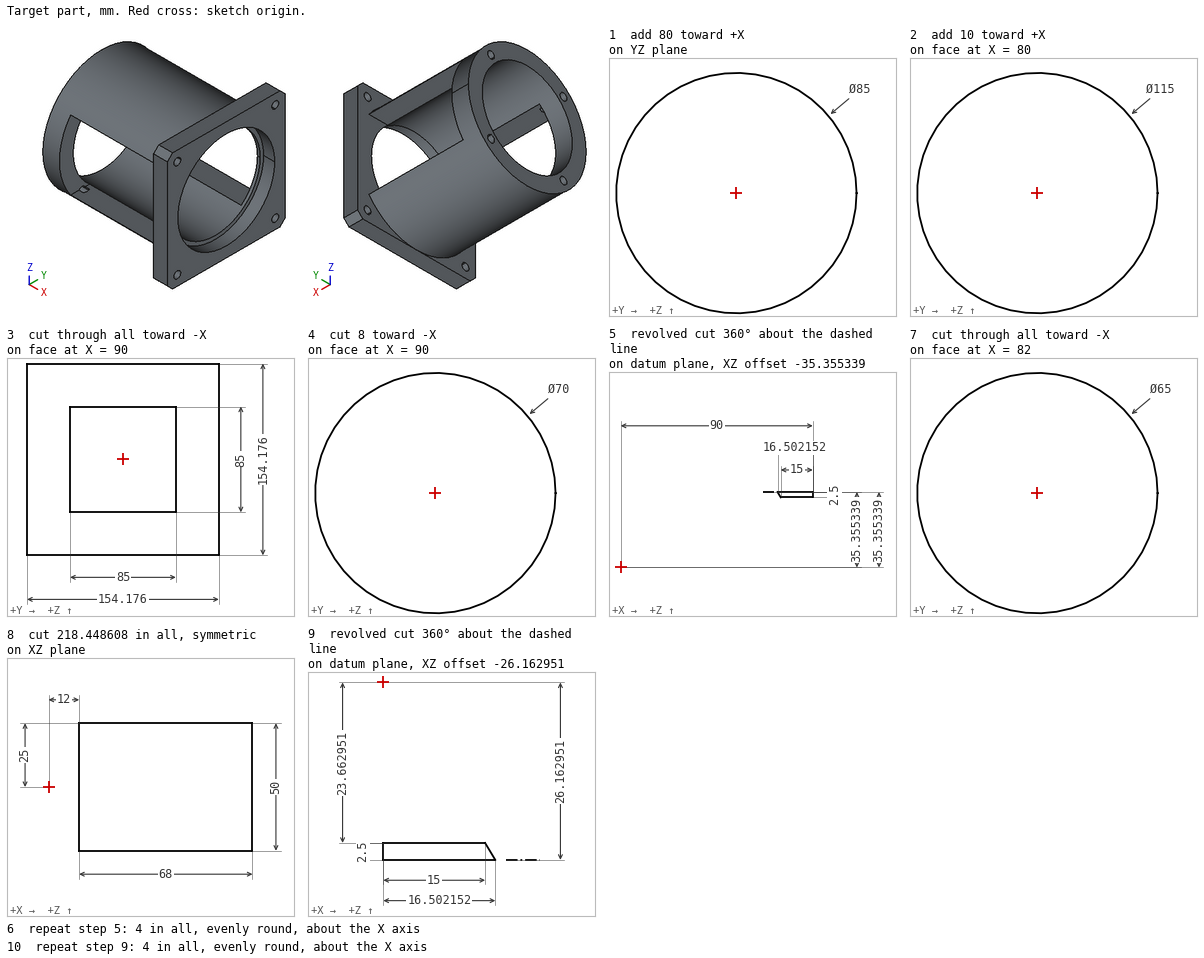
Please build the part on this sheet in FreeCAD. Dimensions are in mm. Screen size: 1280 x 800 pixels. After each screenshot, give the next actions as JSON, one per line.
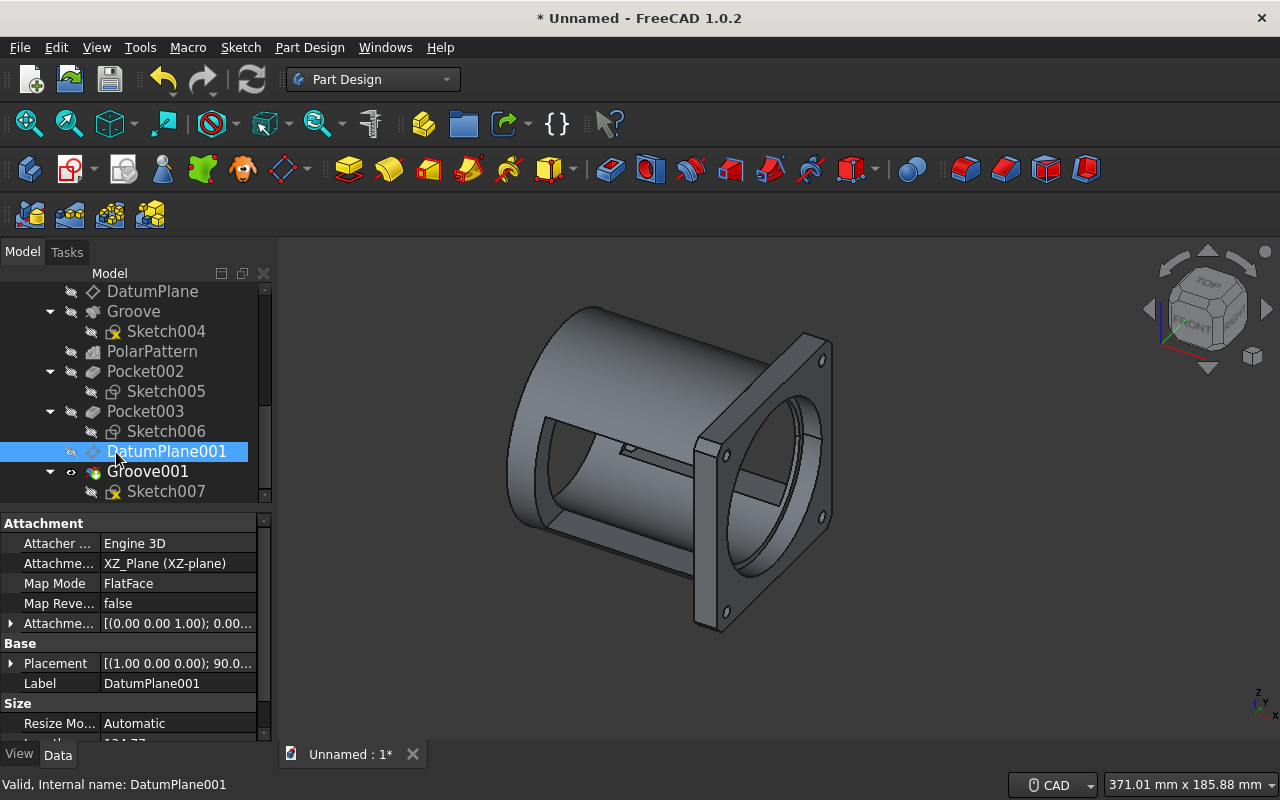
{"action": "left_click", "coordinate": [116, 472]}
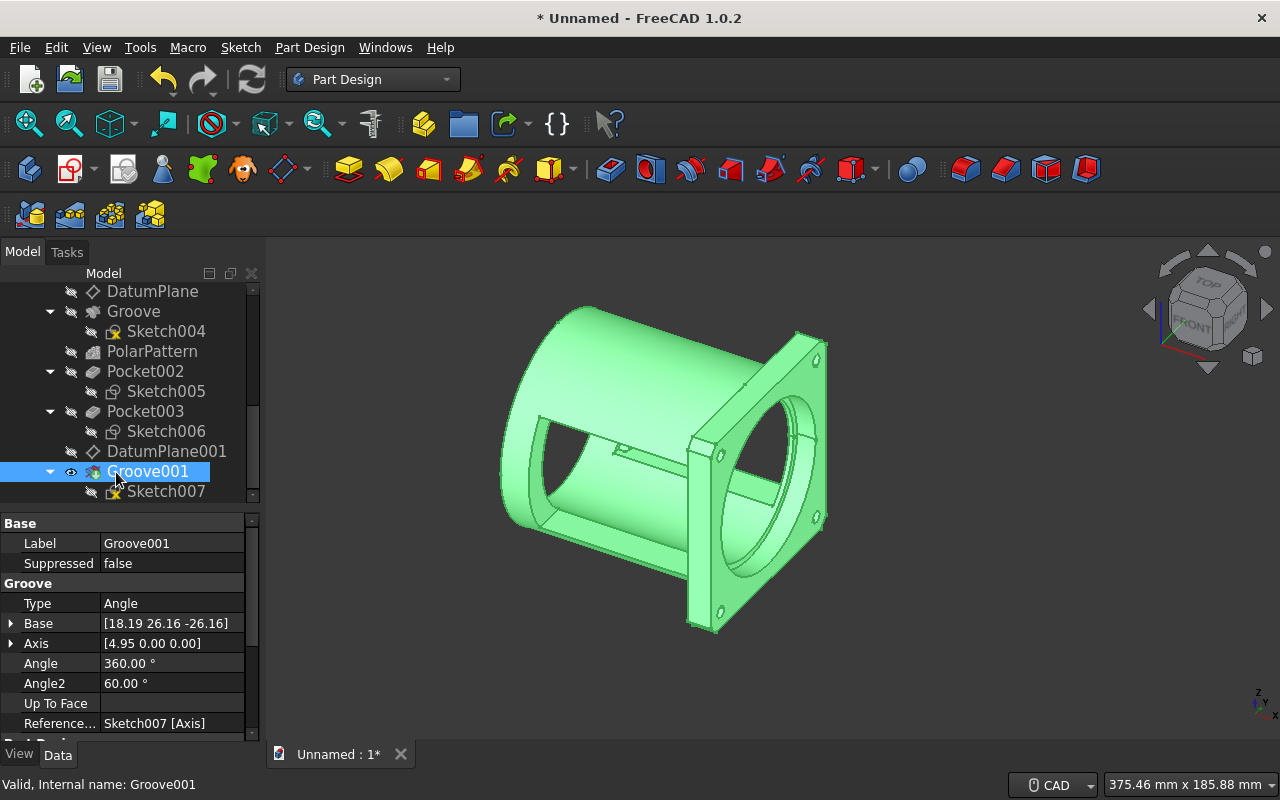
{"action": "left_click", "coordinate": [110, 214]}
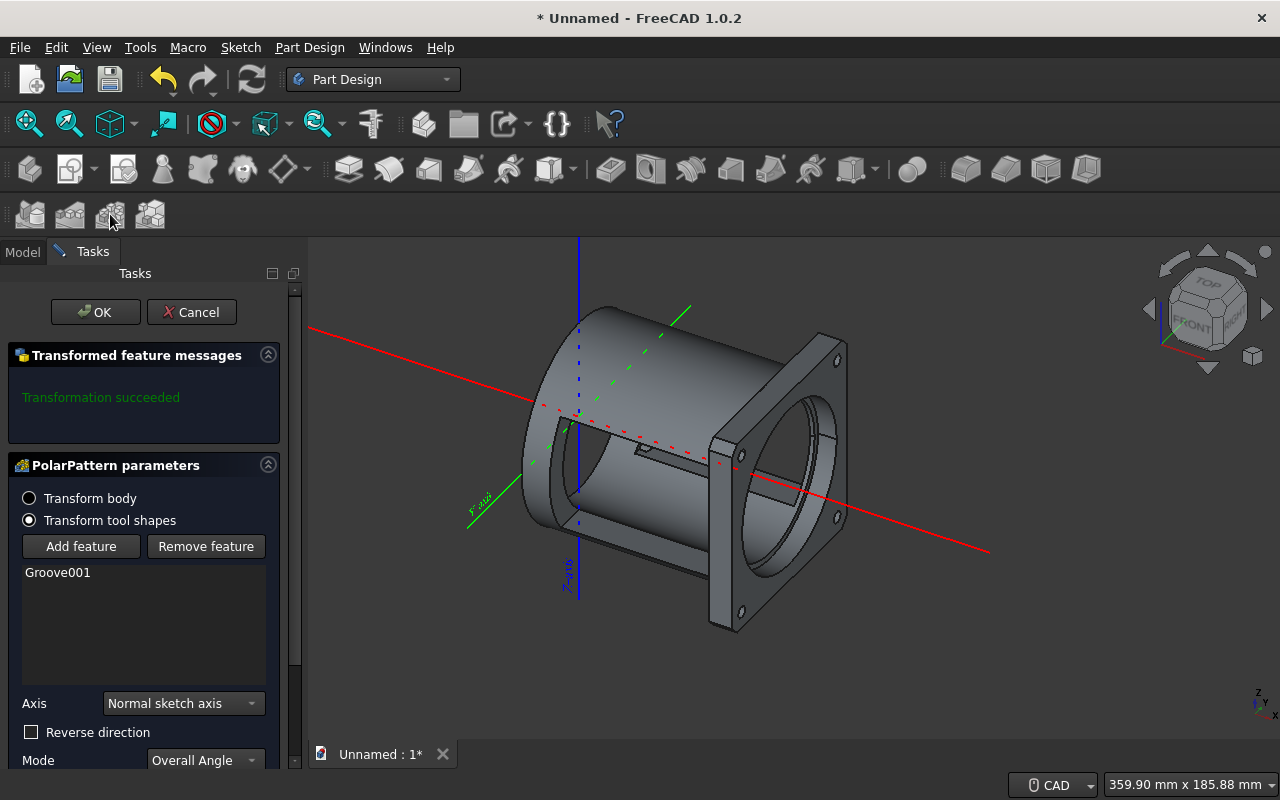
{"action": "left_click", "coordinate": [184, 704]}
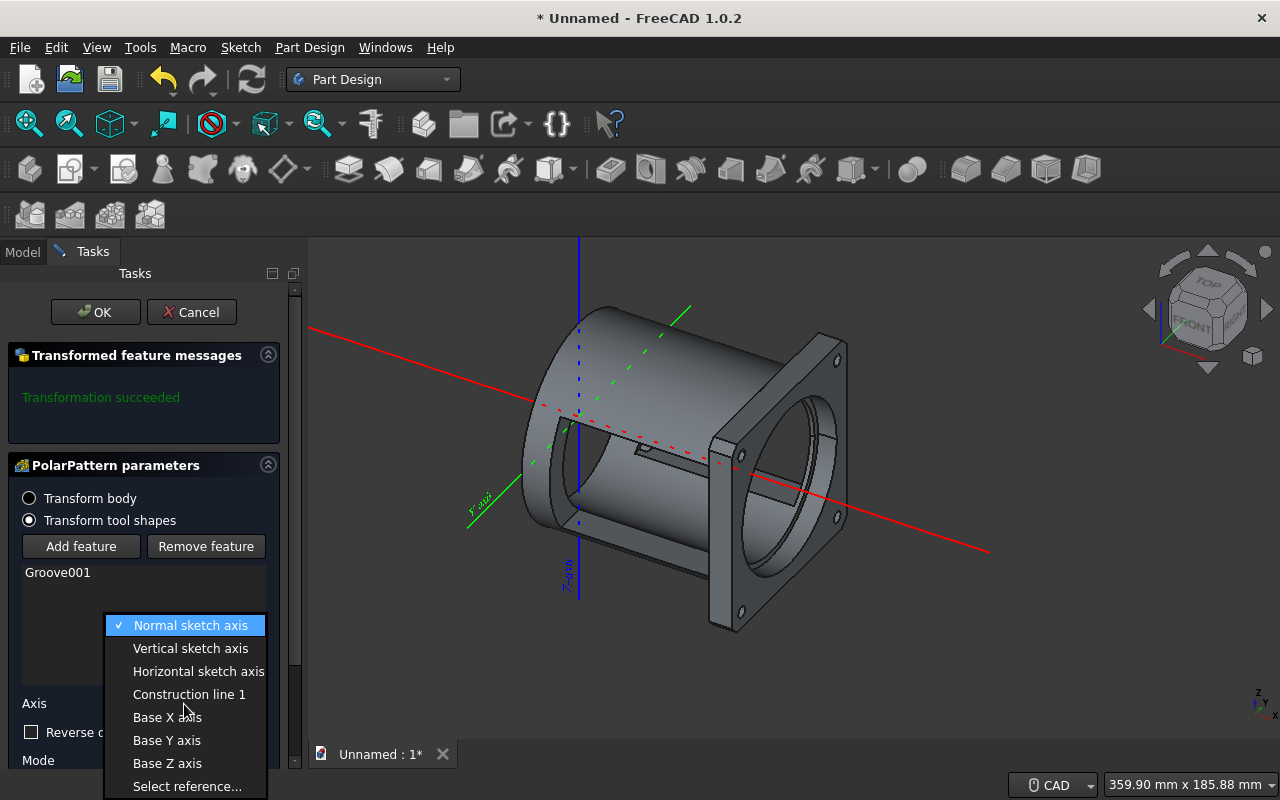
{"action": "left_click", "coordinate": [184, 718]}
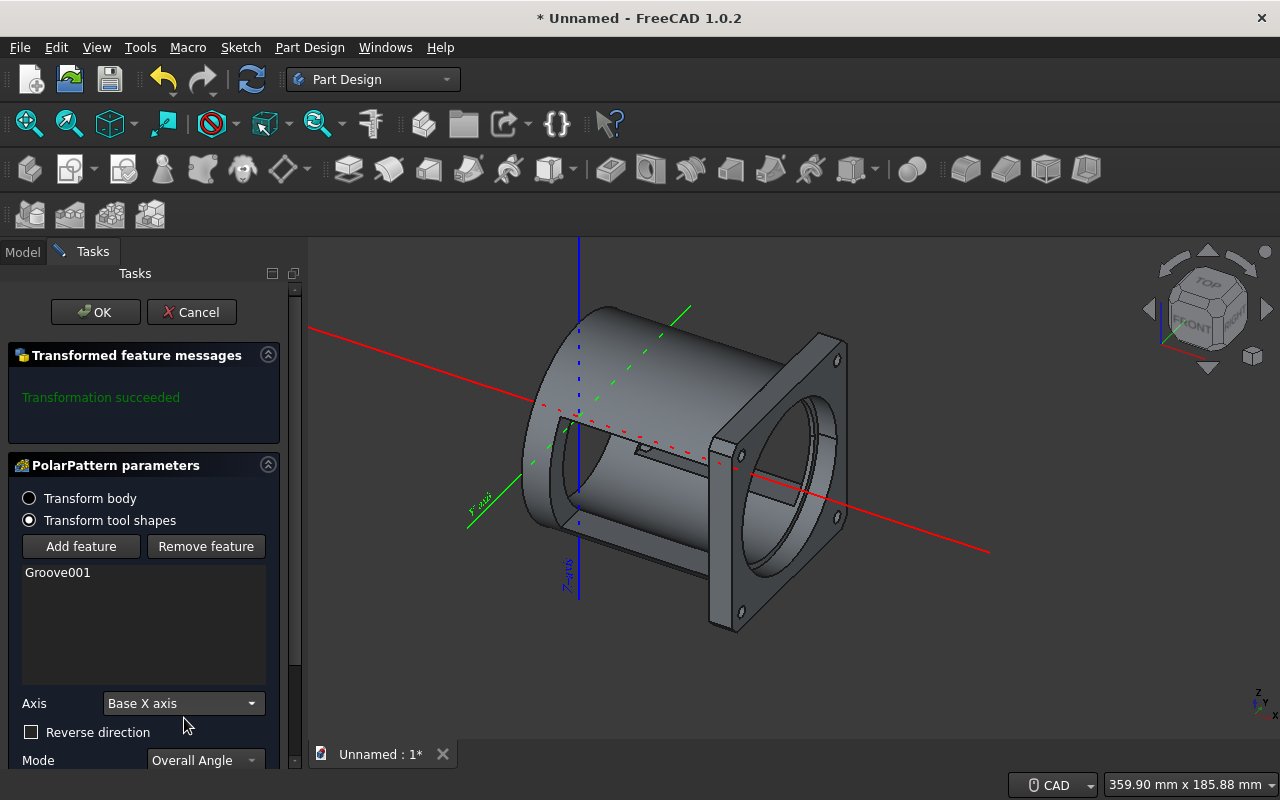
{"action": "scroll", "coordinate": [295, 526], "scroll_direction": "down", "scroll_amount": 3}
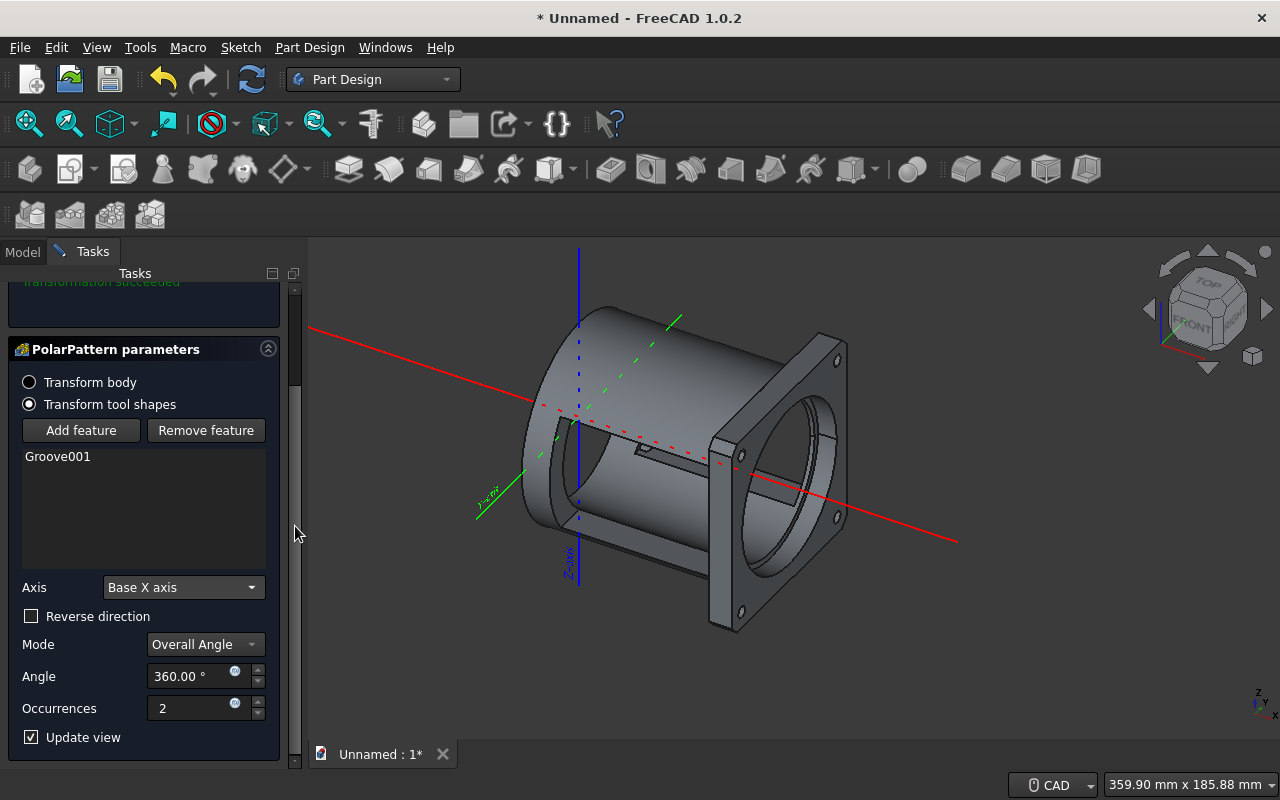
{"action": "triple_click", "coordinate": [198, 708]}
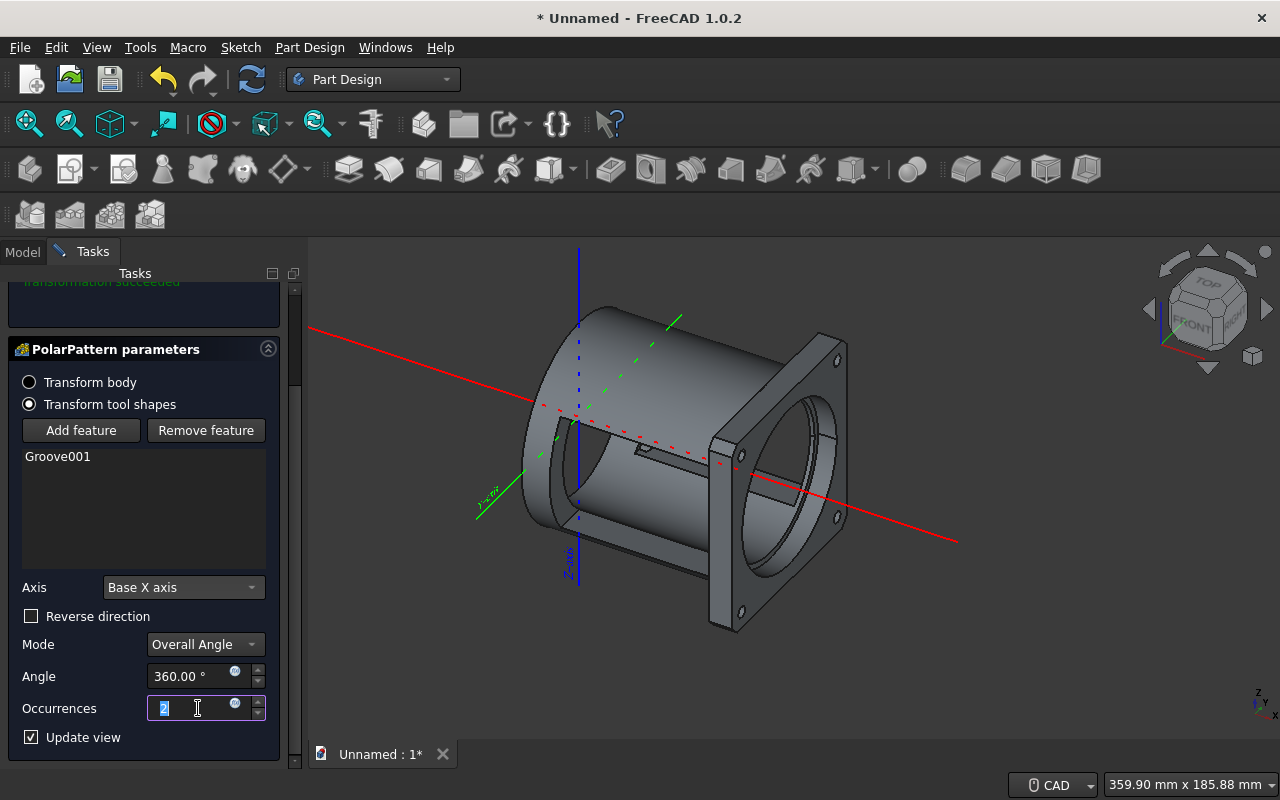
{"action": "type", "text": "4"}
{"action": "key", "text": "Tab"}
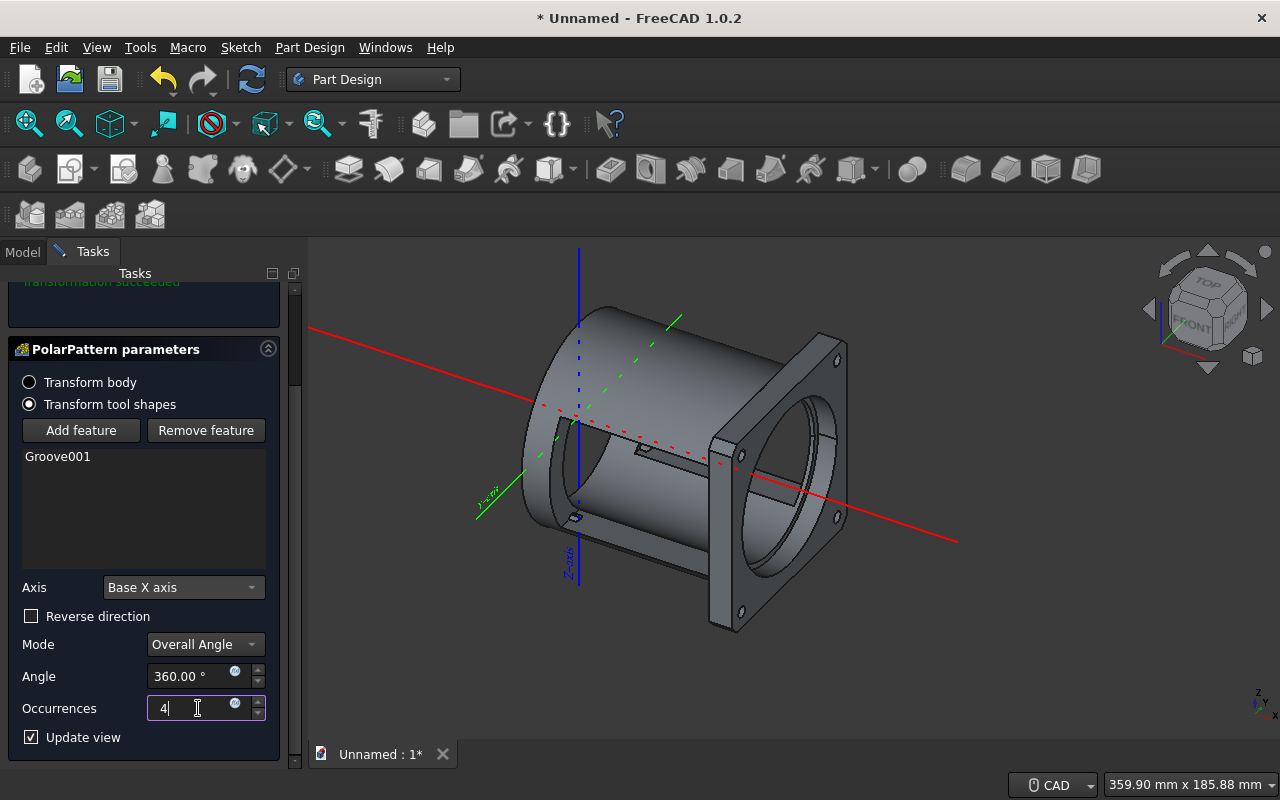
{"action": "scroll", "coordinate": [295, 526], "scroll_direction": "up", "scroll_amount": 3}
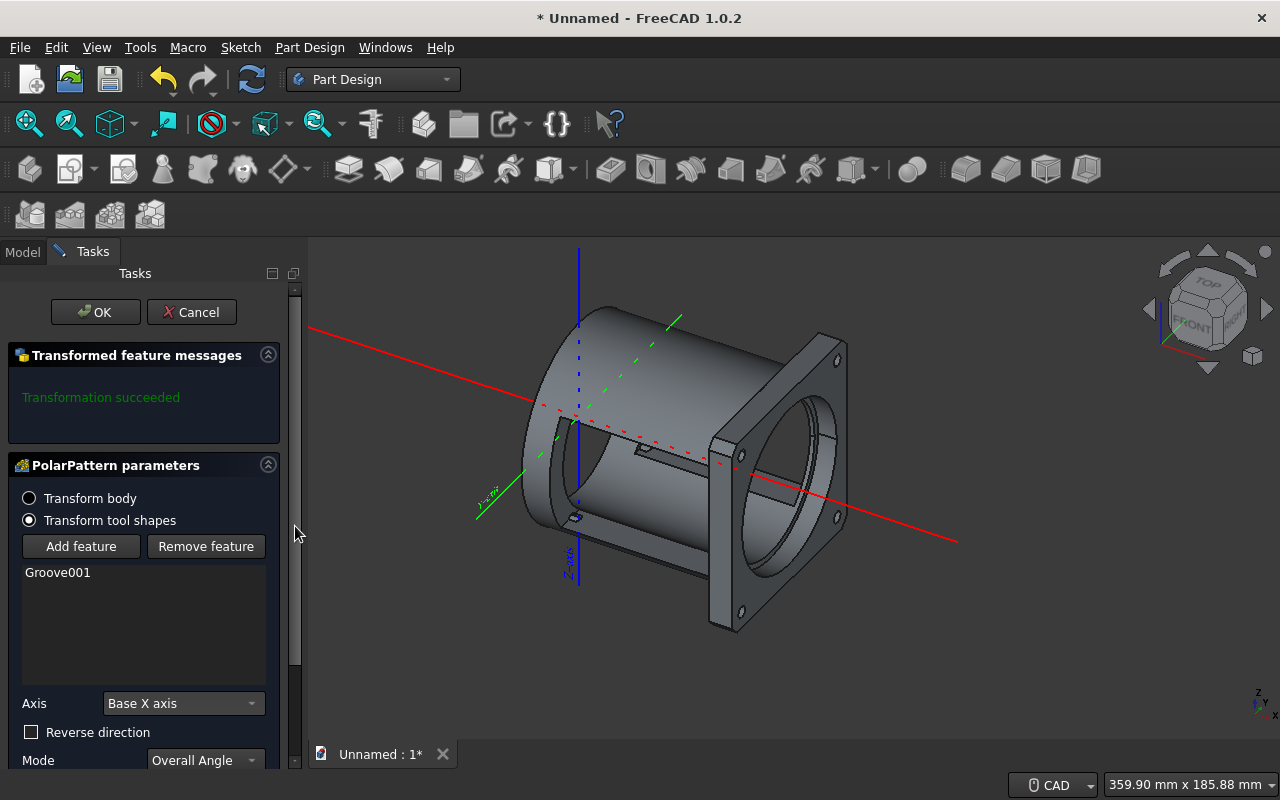
{"action": "left_click", "coordinate": [96, 312]}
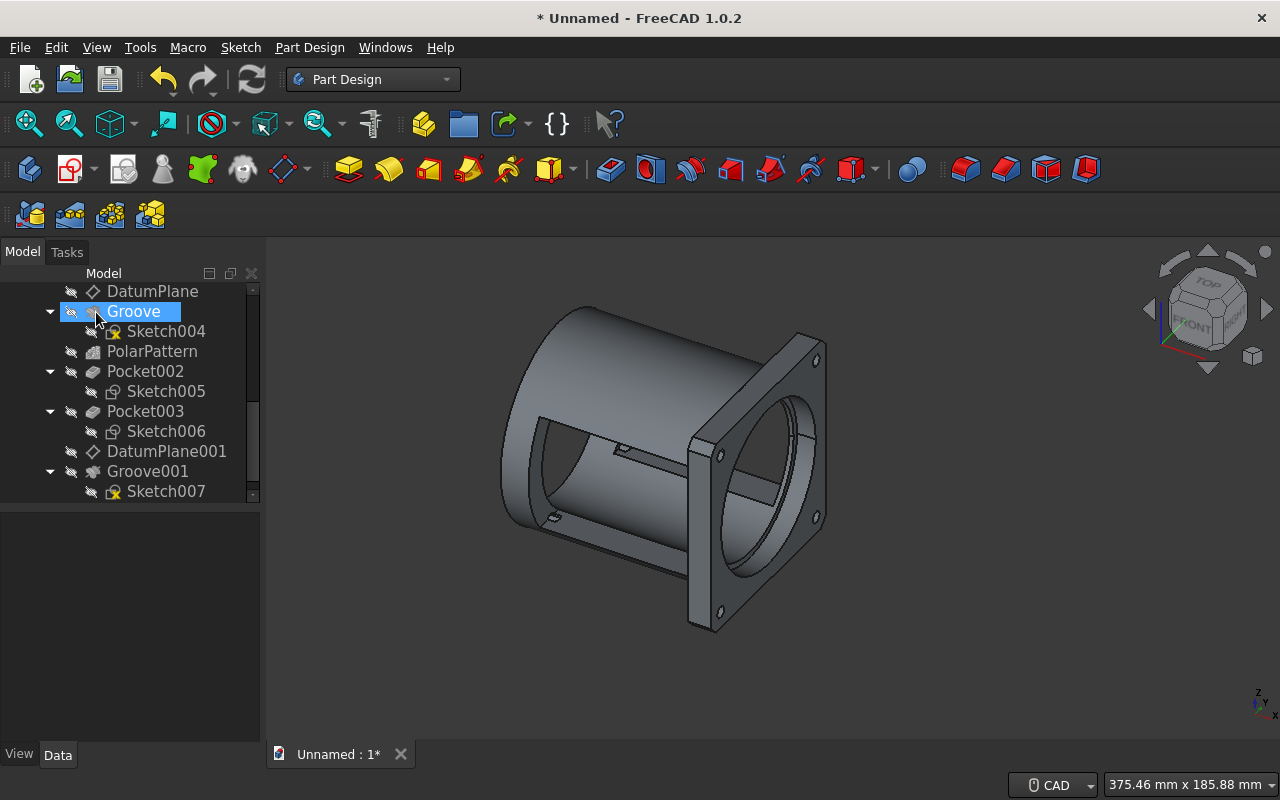
{"action": "key", "text": "0"}